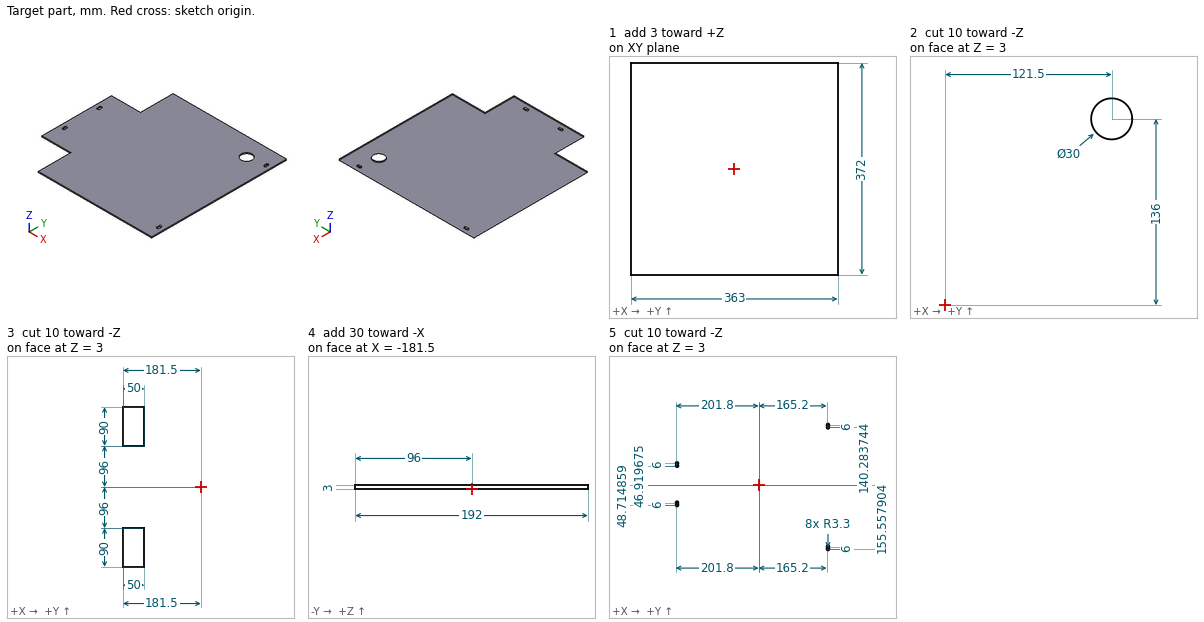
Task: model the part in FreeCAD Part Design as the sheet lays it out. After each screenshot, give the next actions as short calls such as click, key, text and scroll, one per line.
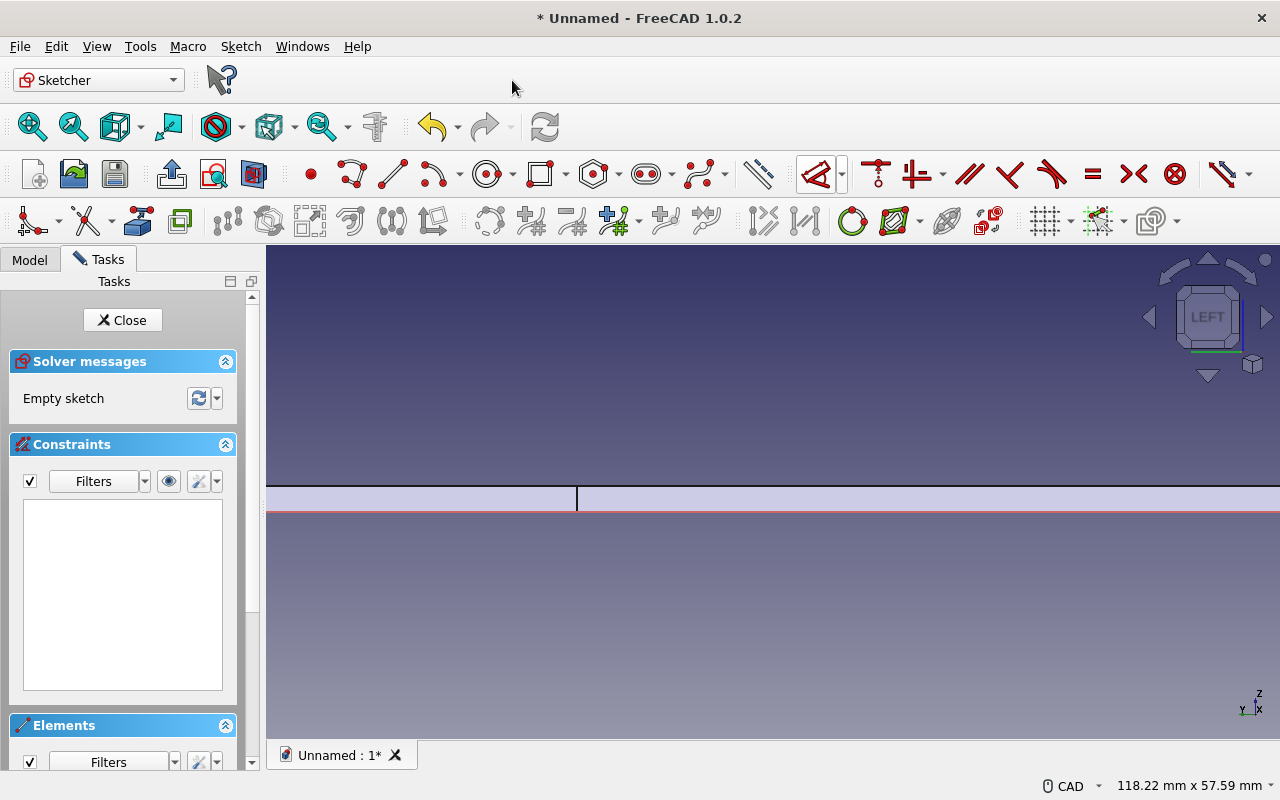
scroll(300, 488, down, 5)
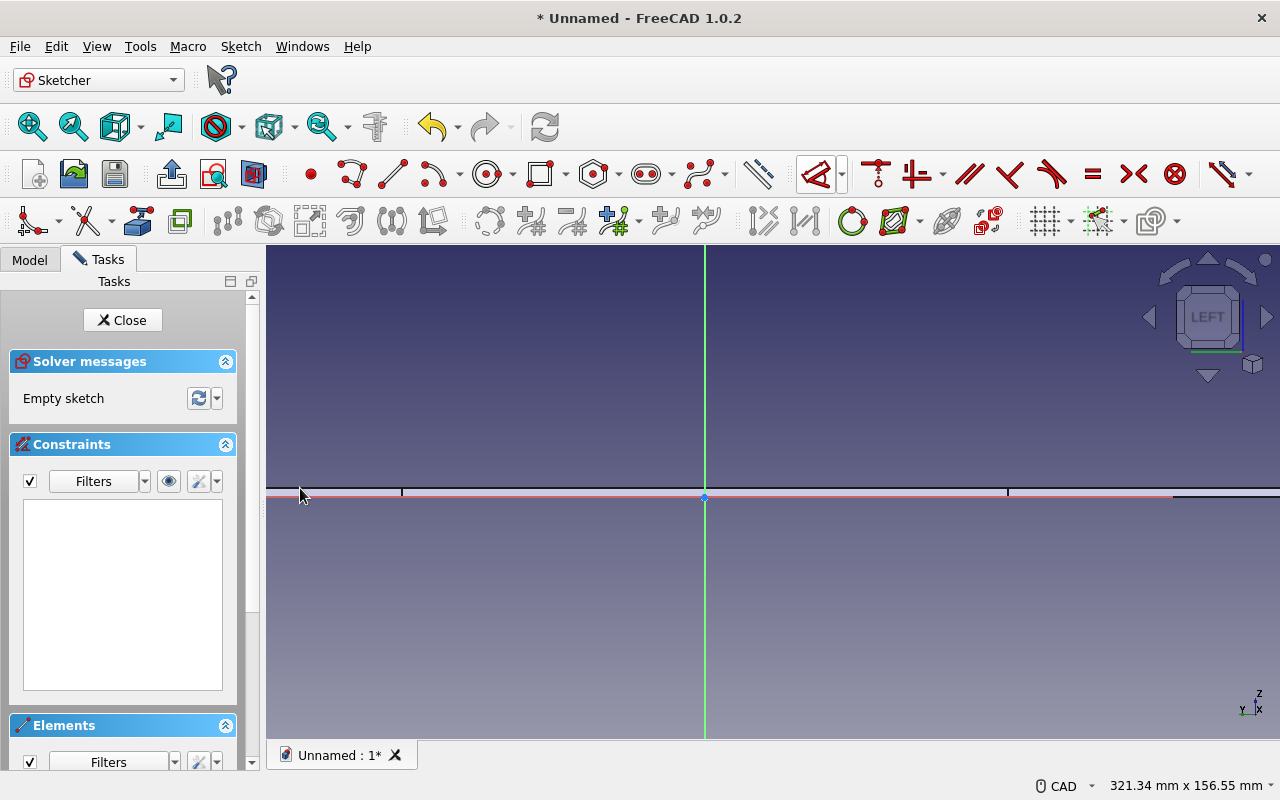
key(g)
key(r)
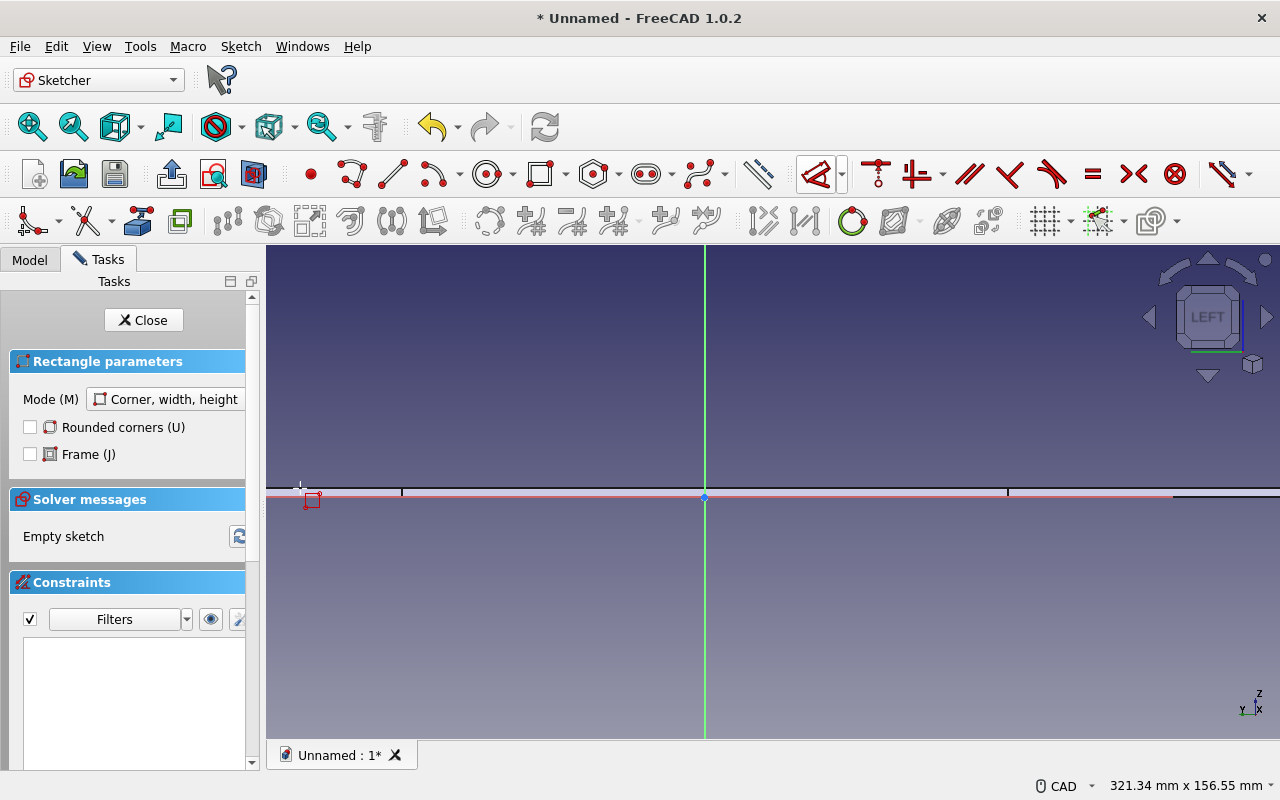
scroll(402, 488, up, 3)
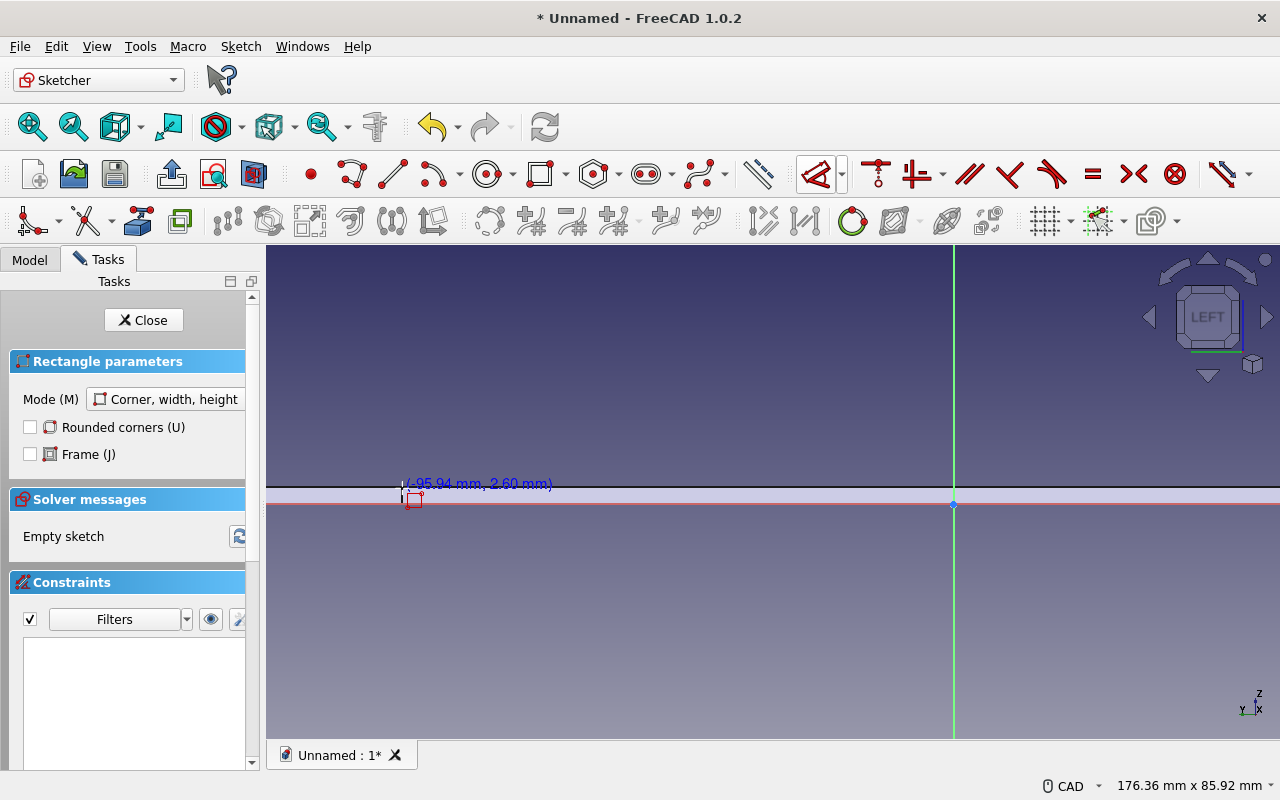
click(402, 487)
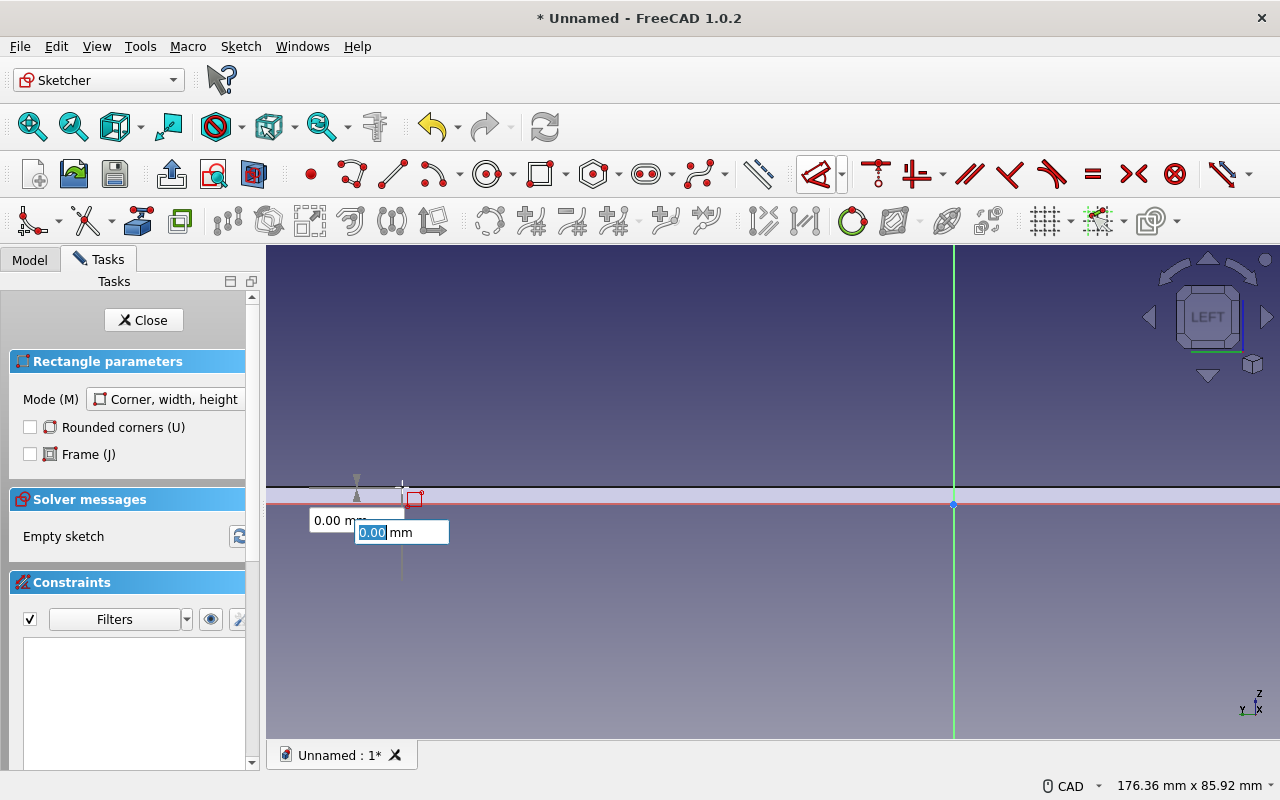
scroll(402, 487, down, 3)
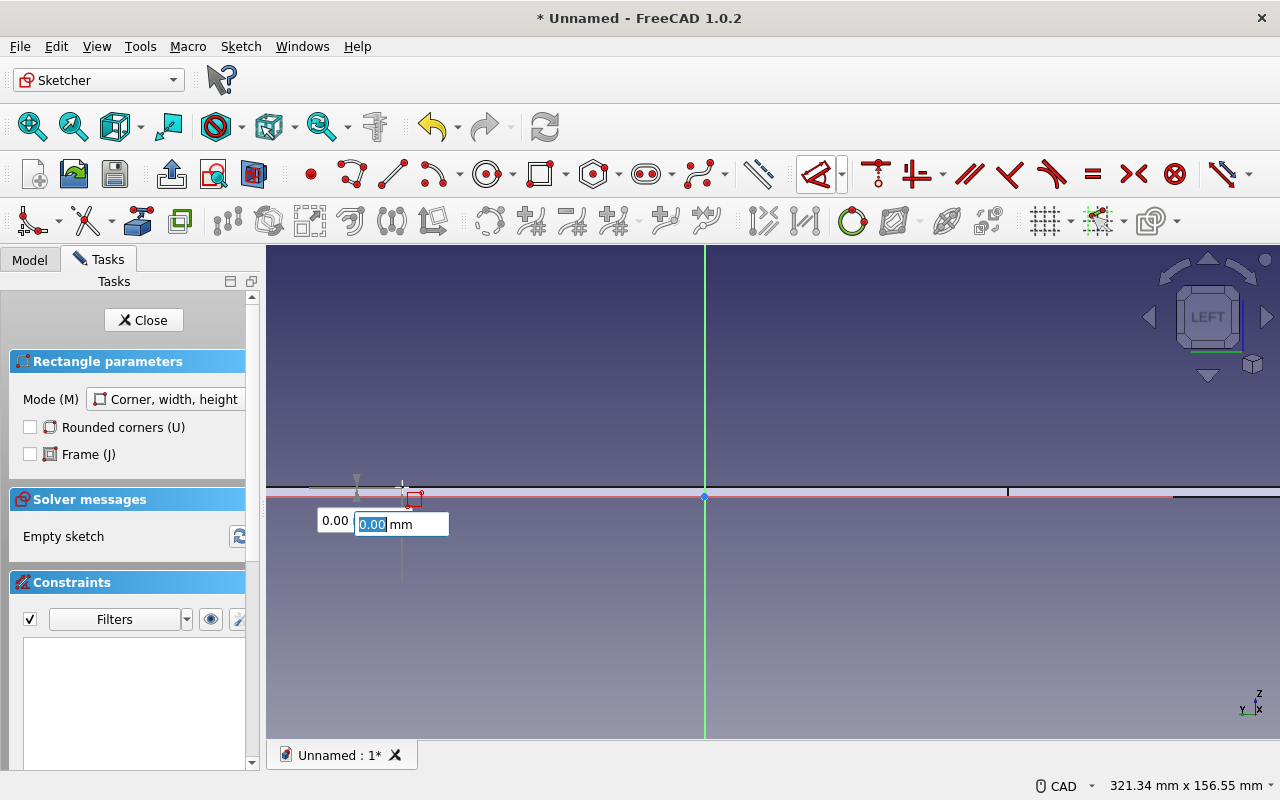
click(1008, 497)
key(Escape)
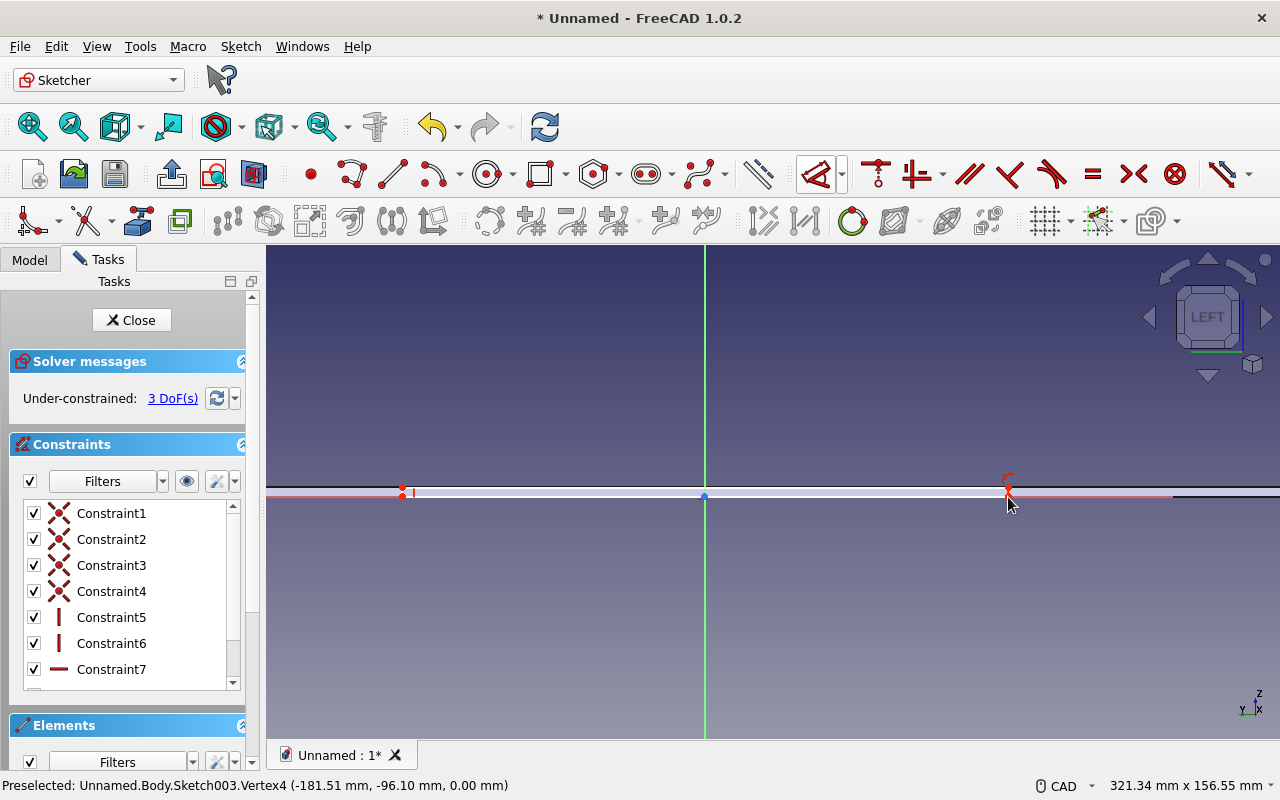
scroll(402, 492, up, 8)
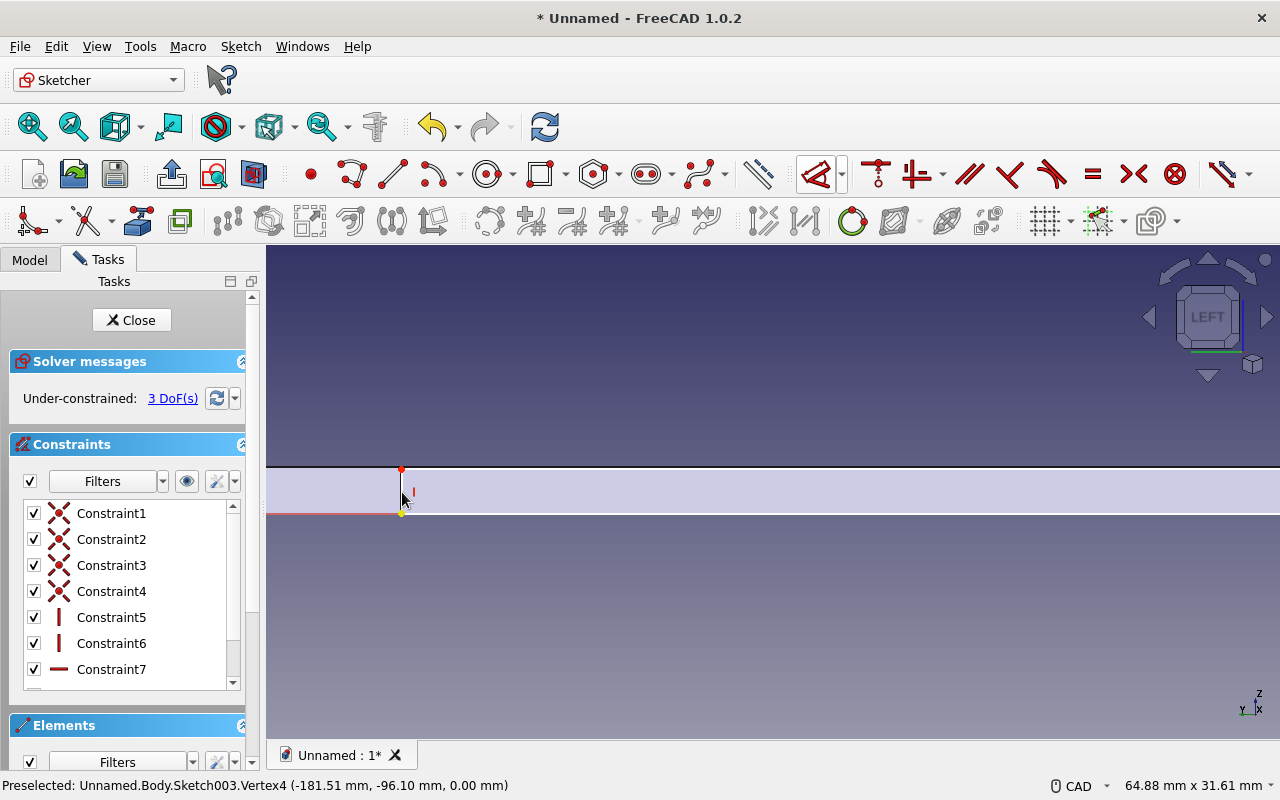
click(402, 491)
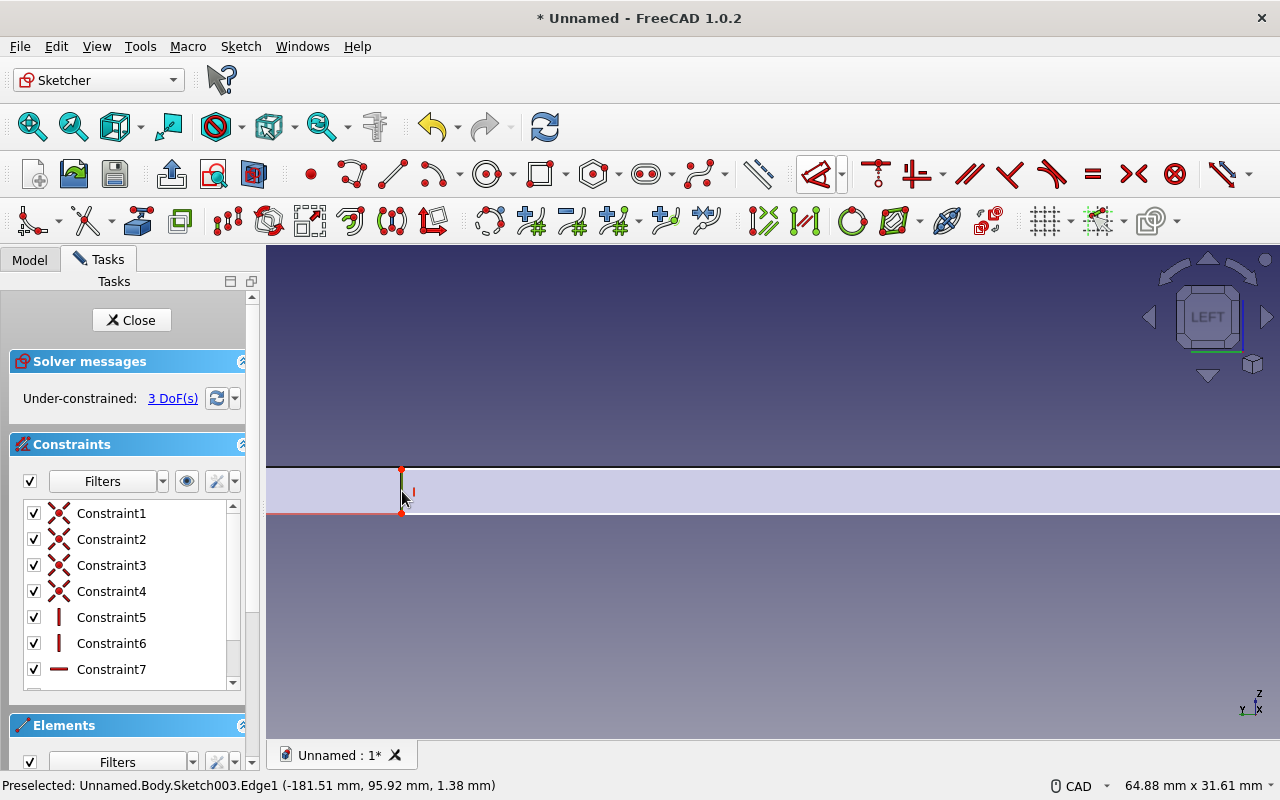
key(i)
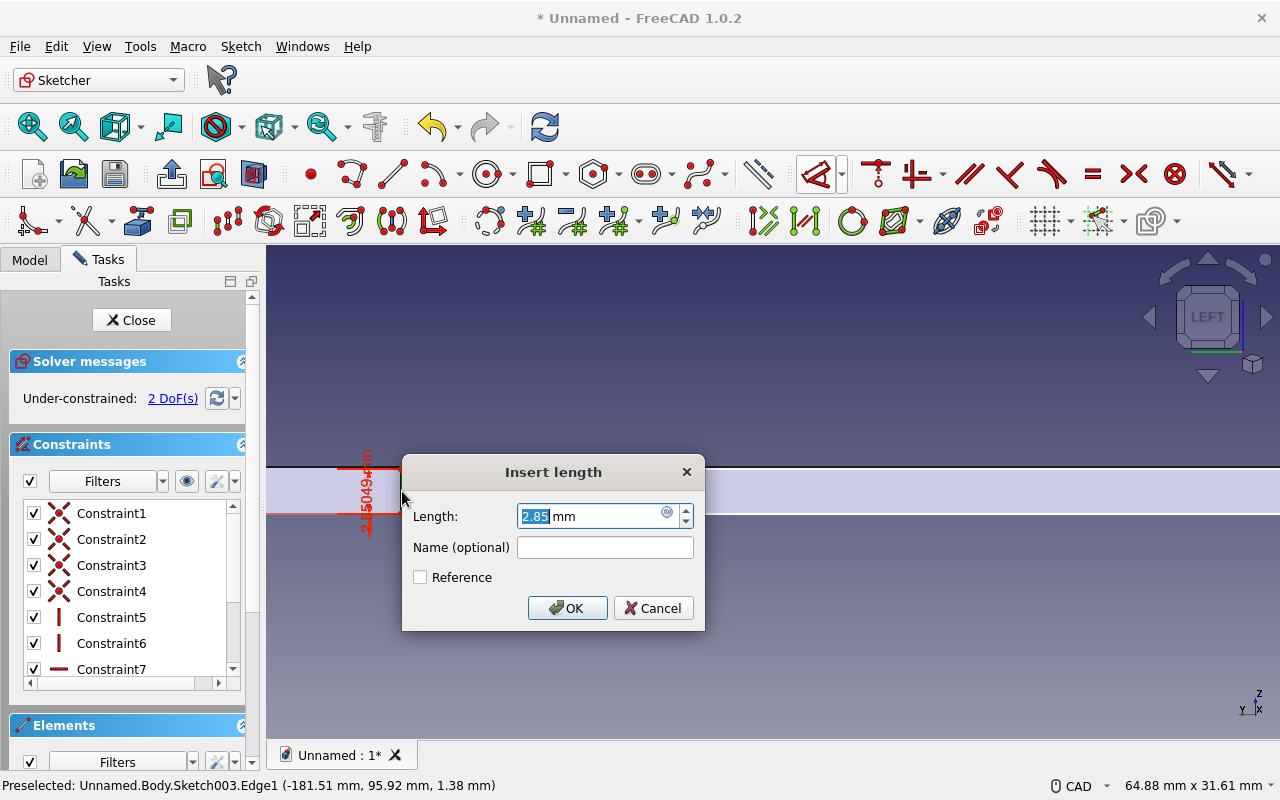
text(3)
key(Return)